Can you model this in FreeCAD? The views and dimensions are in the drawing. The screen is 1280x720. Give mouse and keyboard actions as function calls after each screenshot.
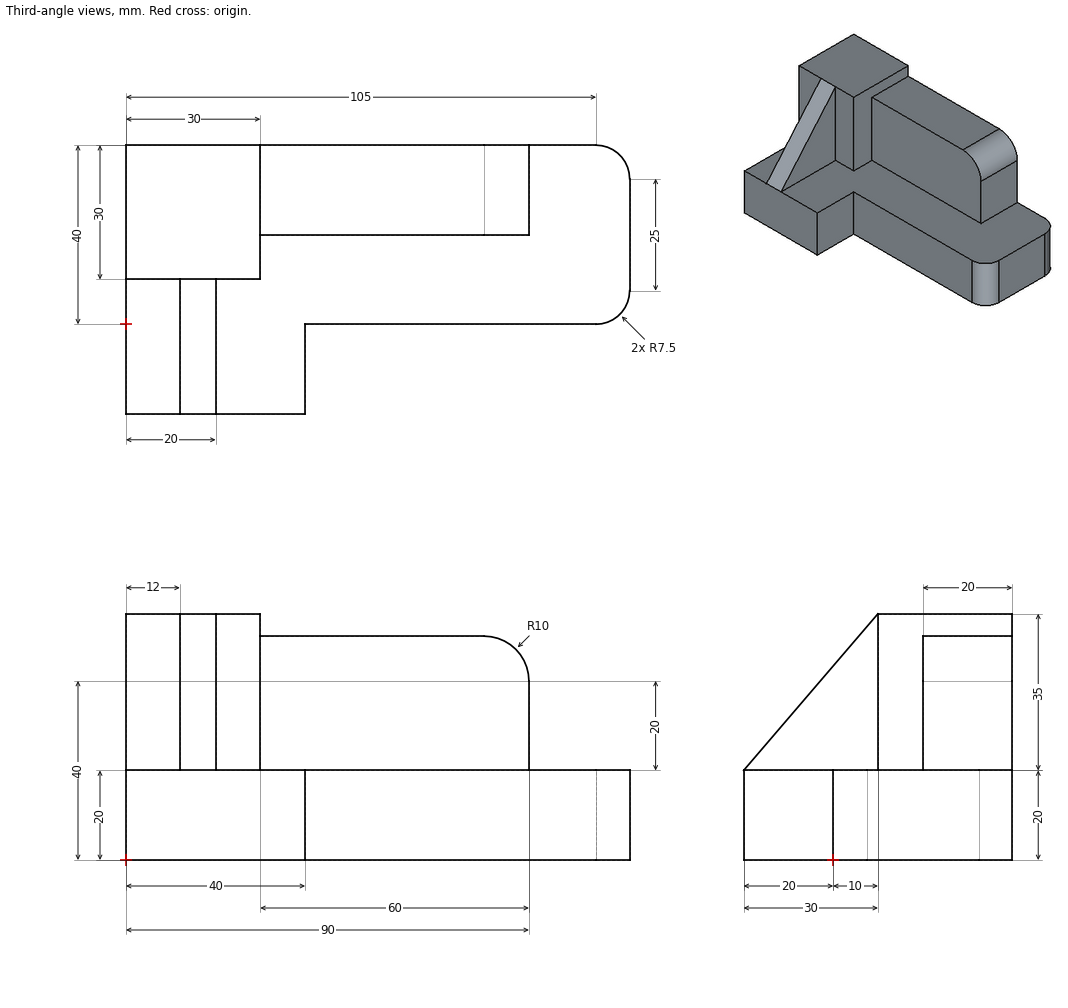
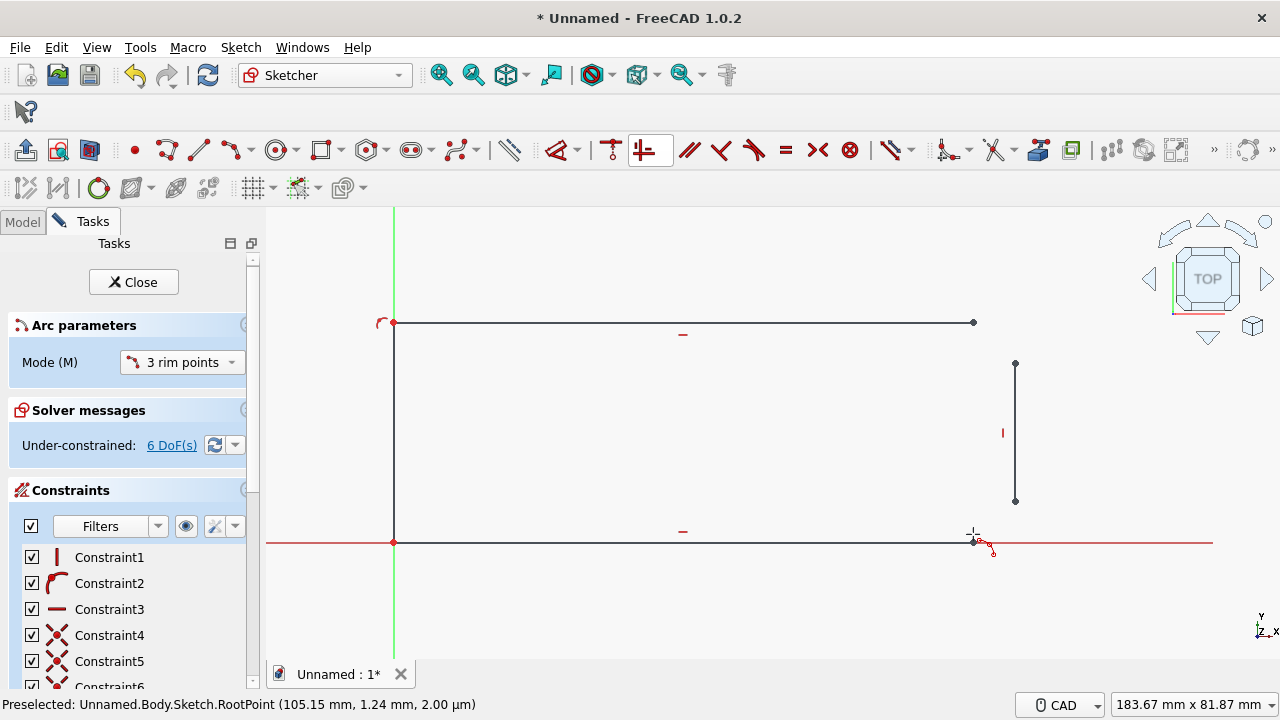
click(1015, 364)
click(973, 323)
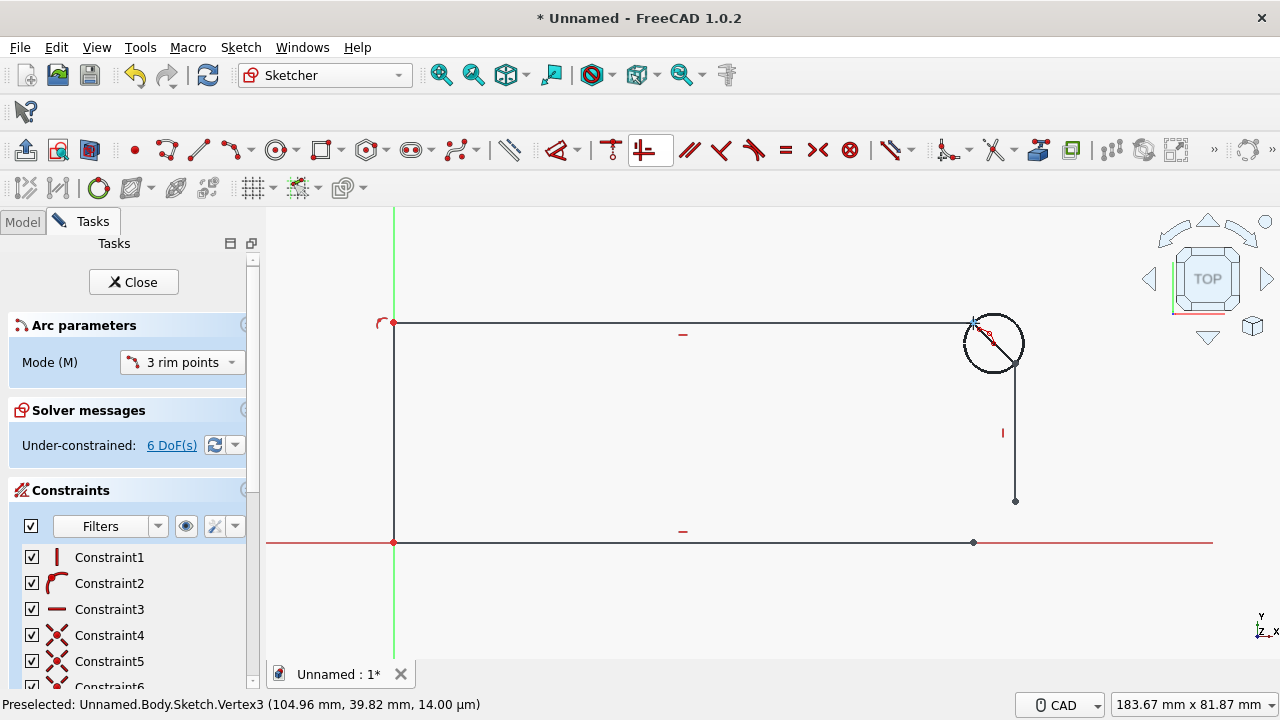
scroll(1002, 334, up, 2)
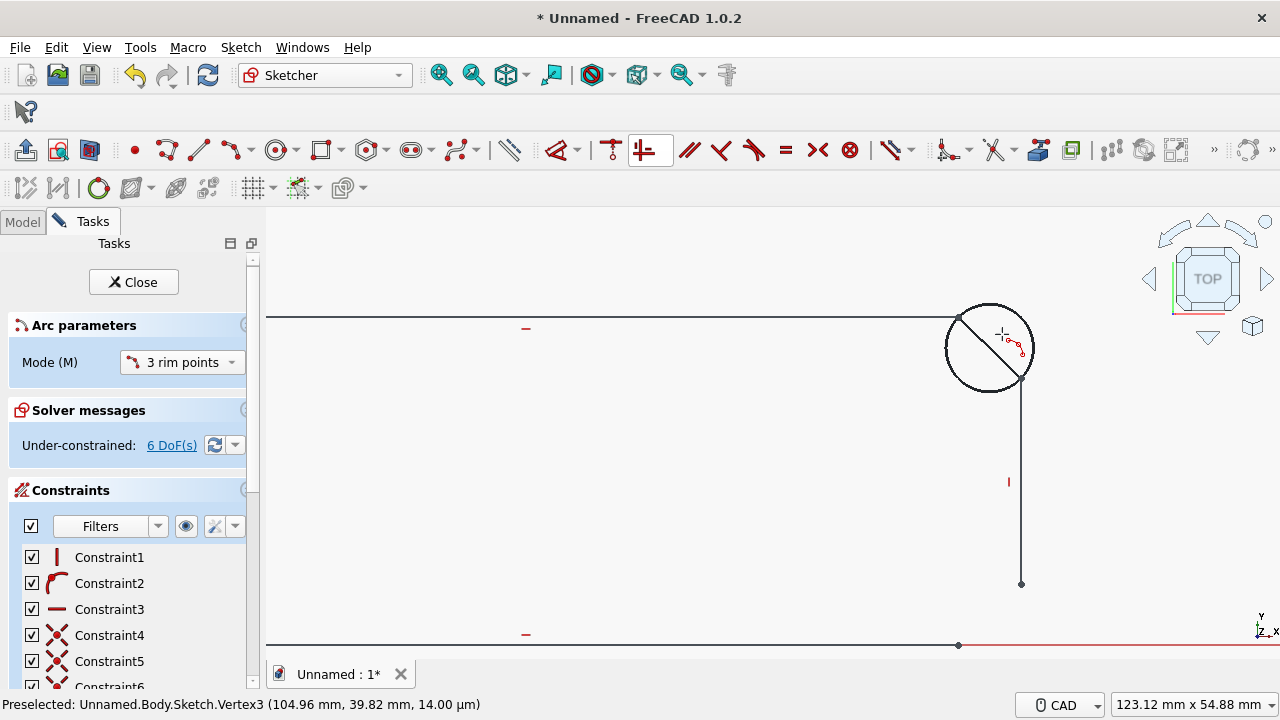
click(1002, 334)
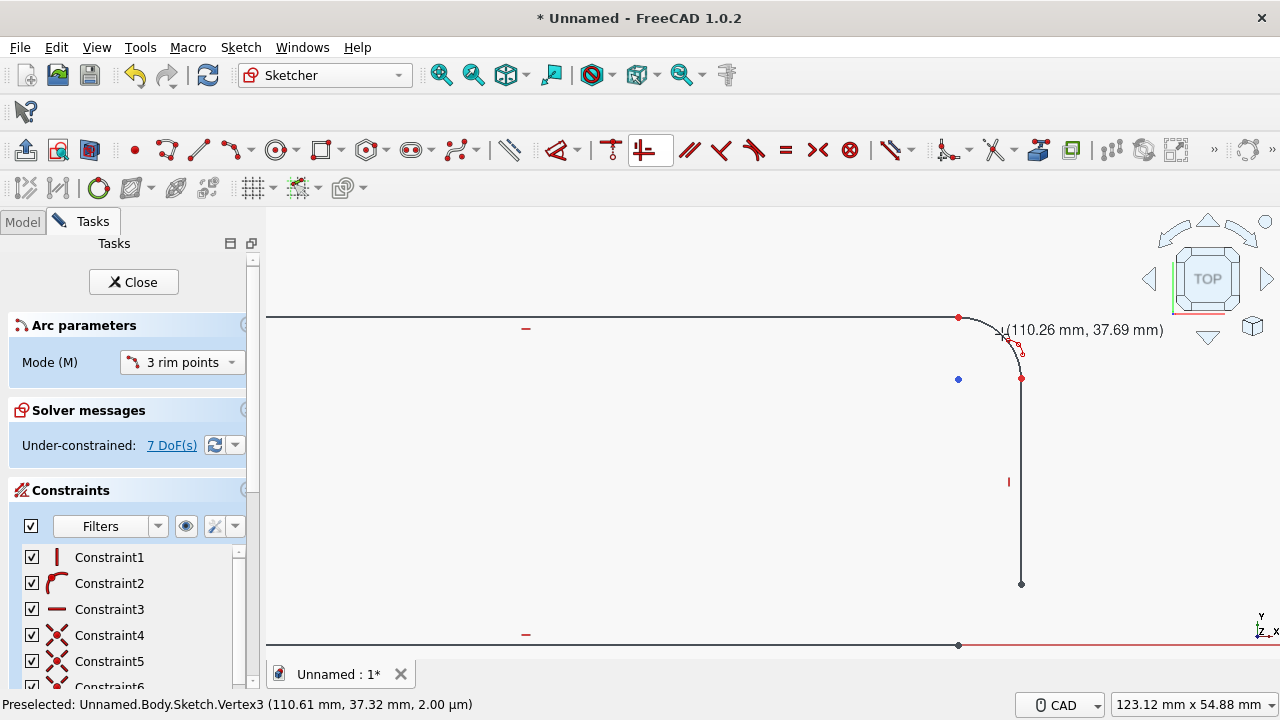
scroll(1004, 336, down, 2)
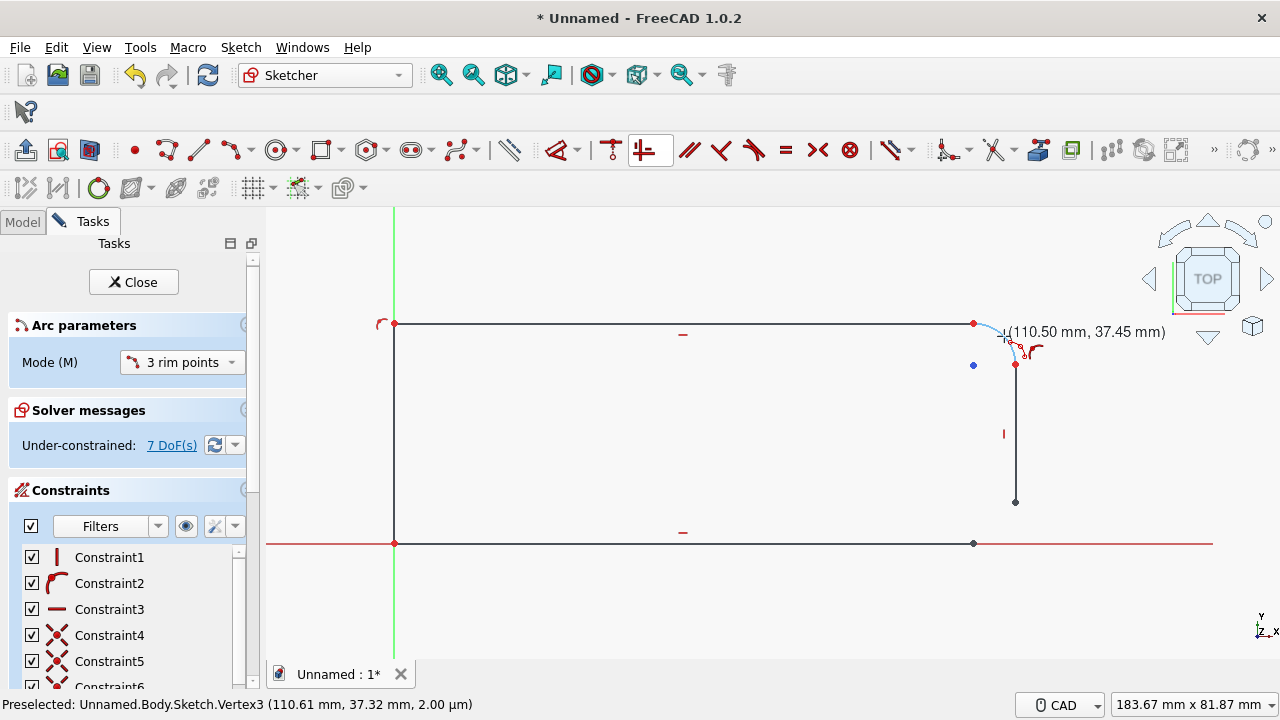
click(974, 544)
click(1016, 503)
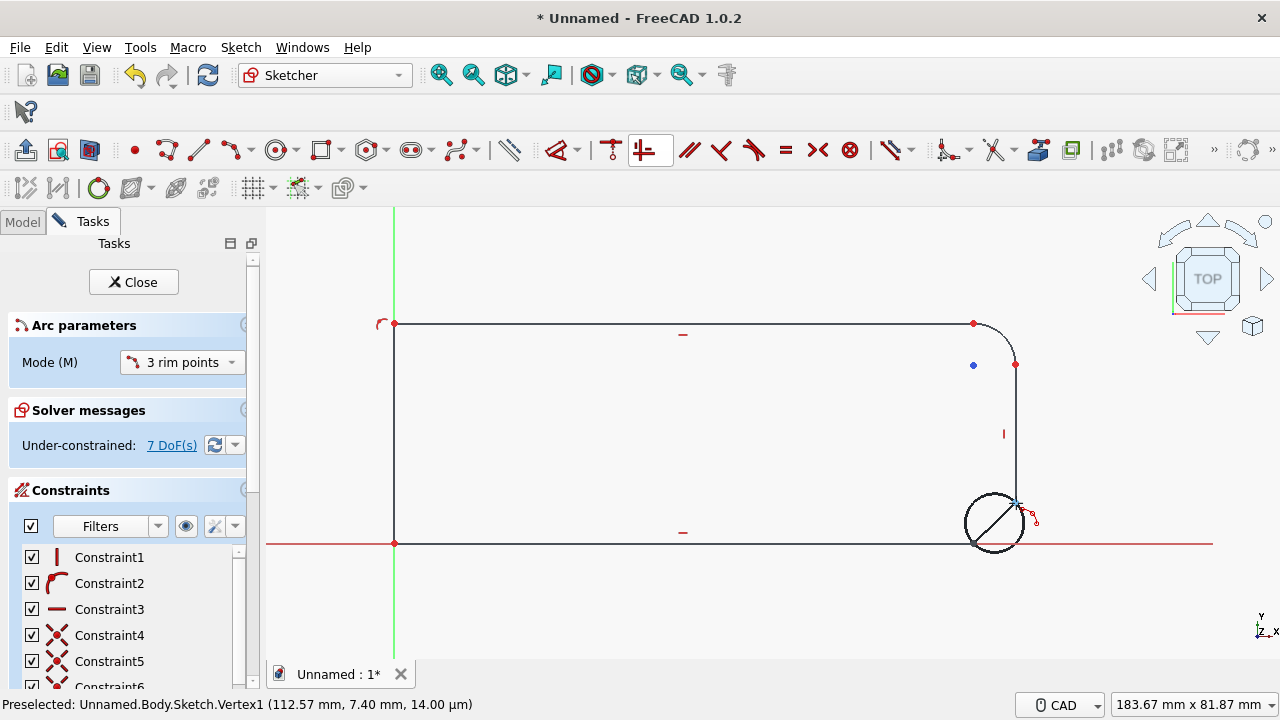
scroll(1003, 531, up, 2)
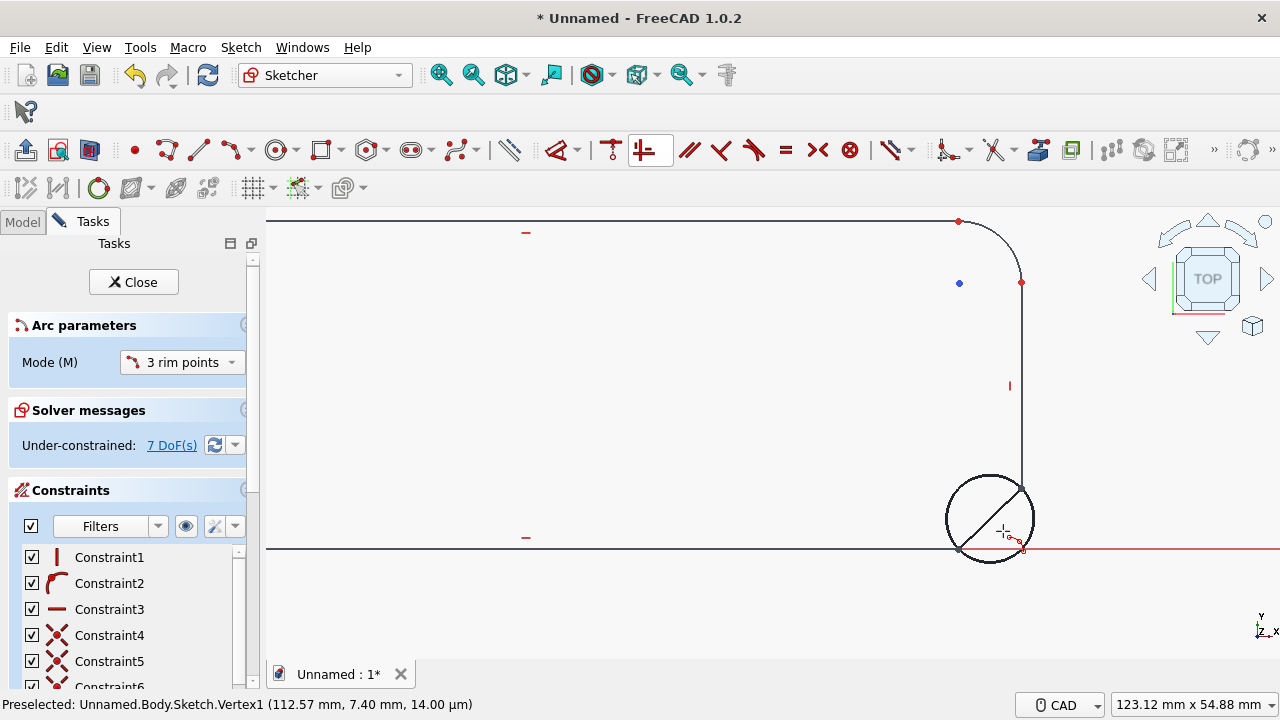
click(1003, 531)
key(Escape)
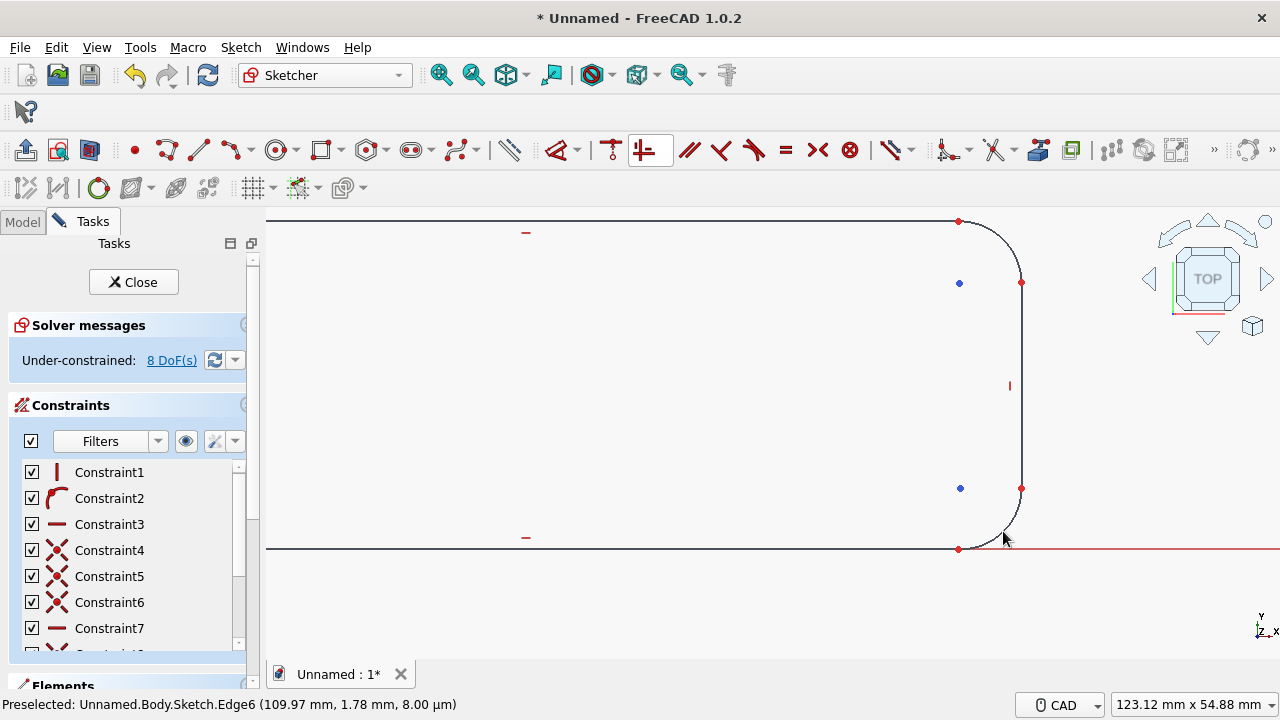
click(1022, 427)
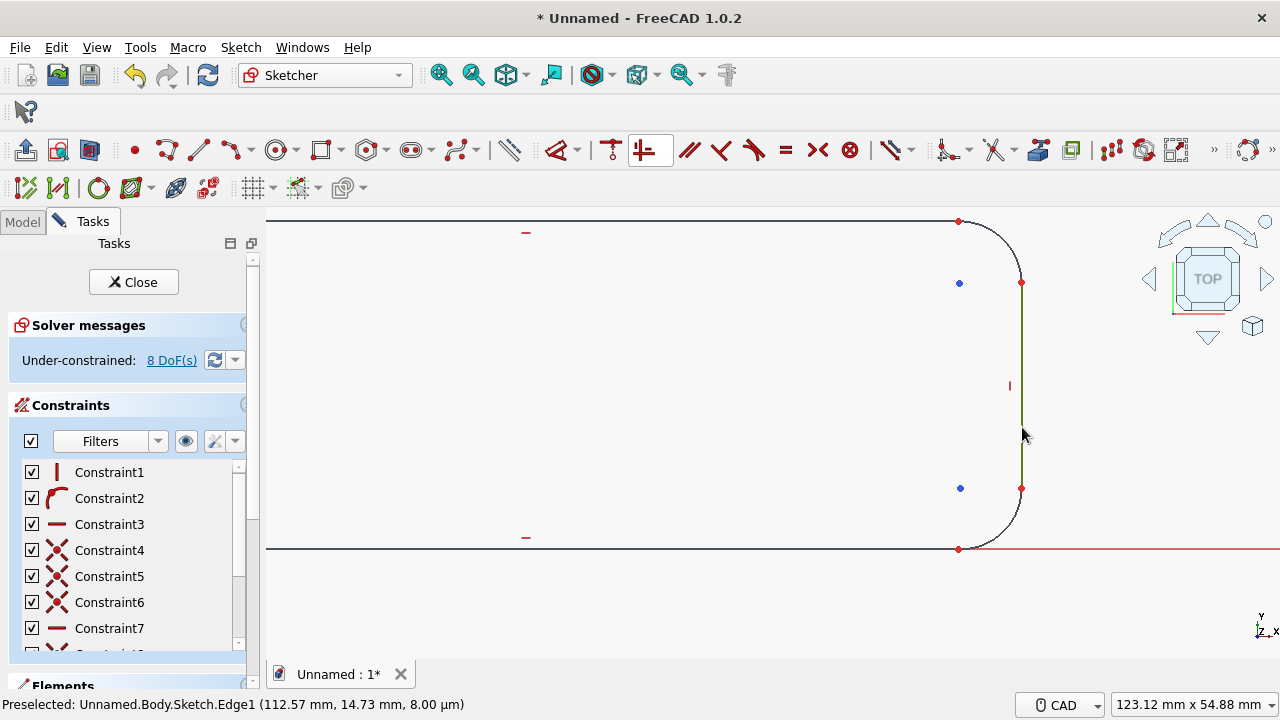
click(1014, 255)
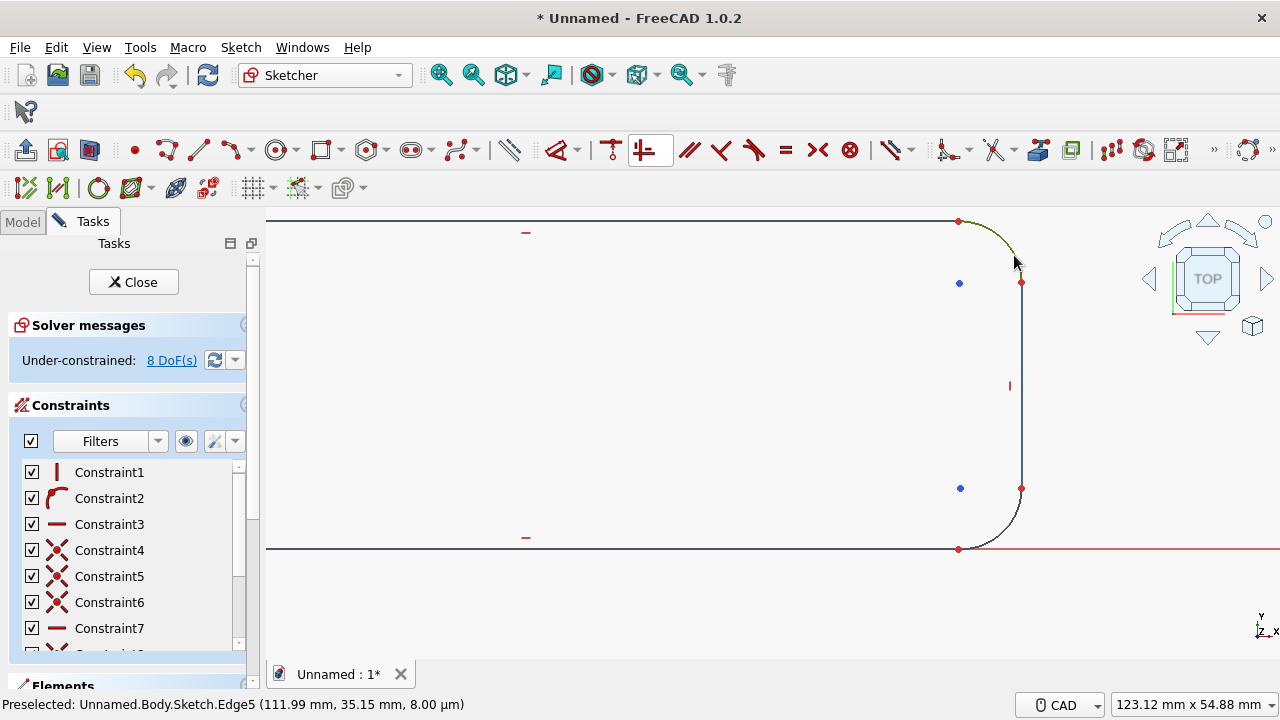
key(t)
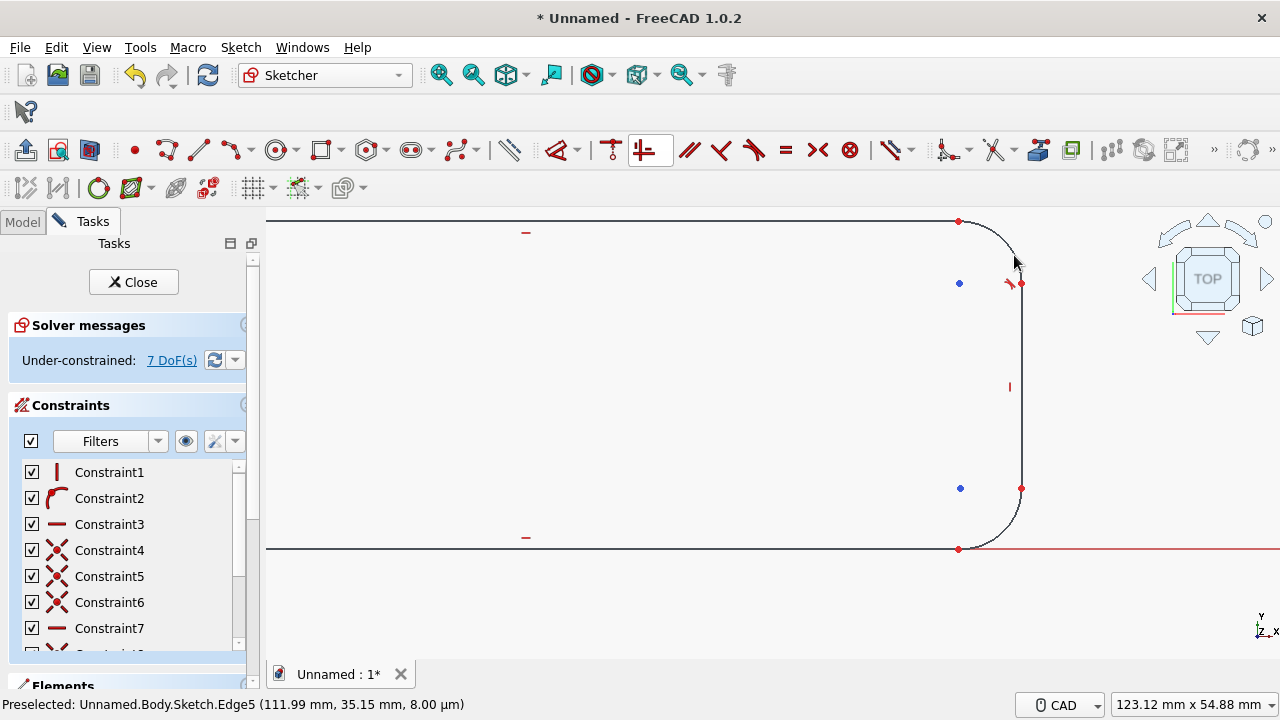
click(1022, 427)